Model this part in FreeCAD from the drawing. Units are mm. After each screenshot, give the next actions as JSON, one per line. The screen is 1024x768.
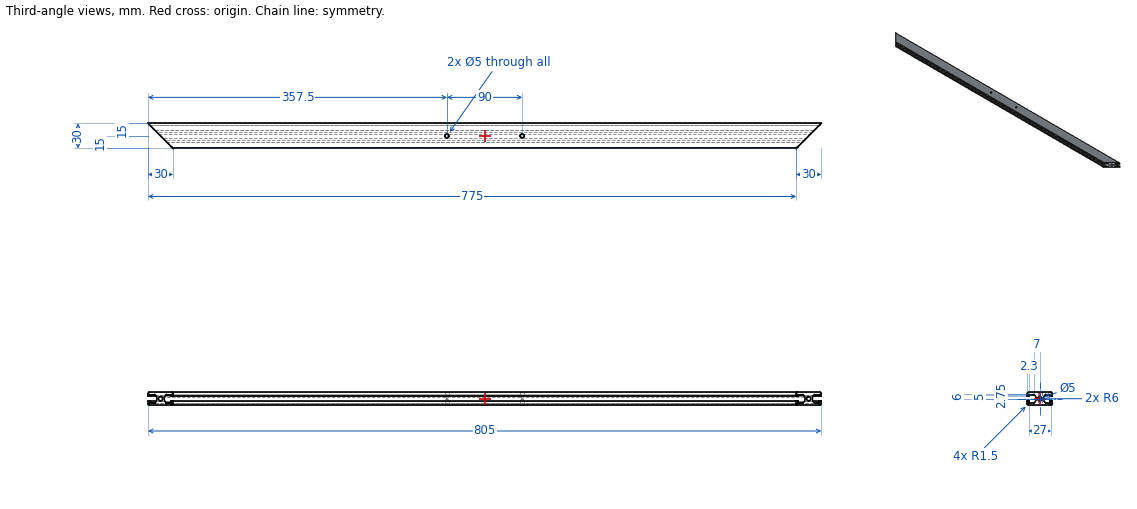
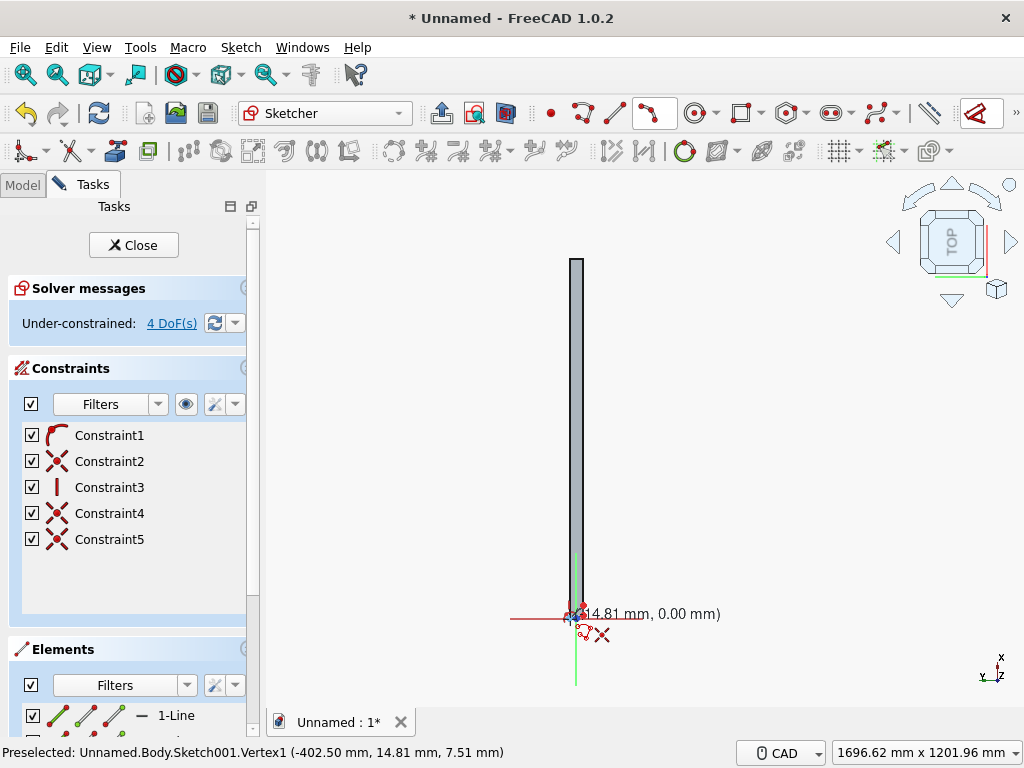
{"action": "scroll", "coordinate": [583, 273], "scroll_direction": "up", "scroll_amount": 5}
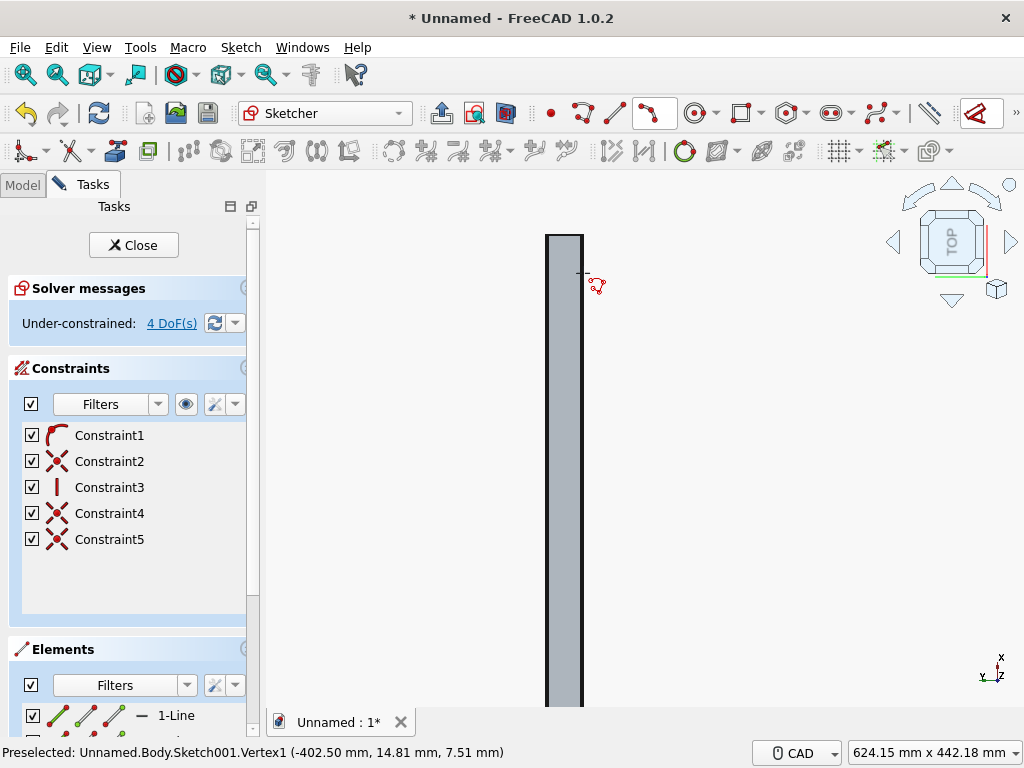
{"action": "left_click", "coordinate": [583, 272]}
{"action": "left_click", "coordinate": [583, 235]}
{"action": "left_click", "coordinate": [546, 235]}
{"action": "left_click", "coordinate": [583, 273]}
{"action": "key", "text": "Escape"}
{"action": "key", "text": "Escape"}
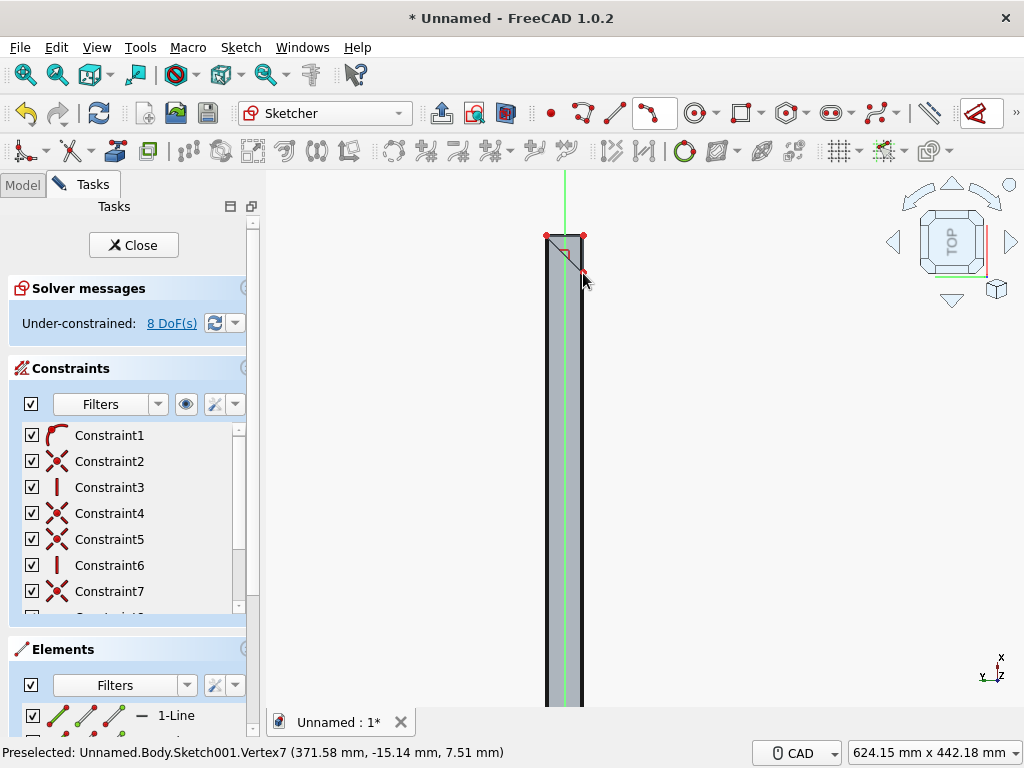
{"action": "scroll", "coordinate": [583, 272], "scroll_direction": "down", "scroll_amount": 5}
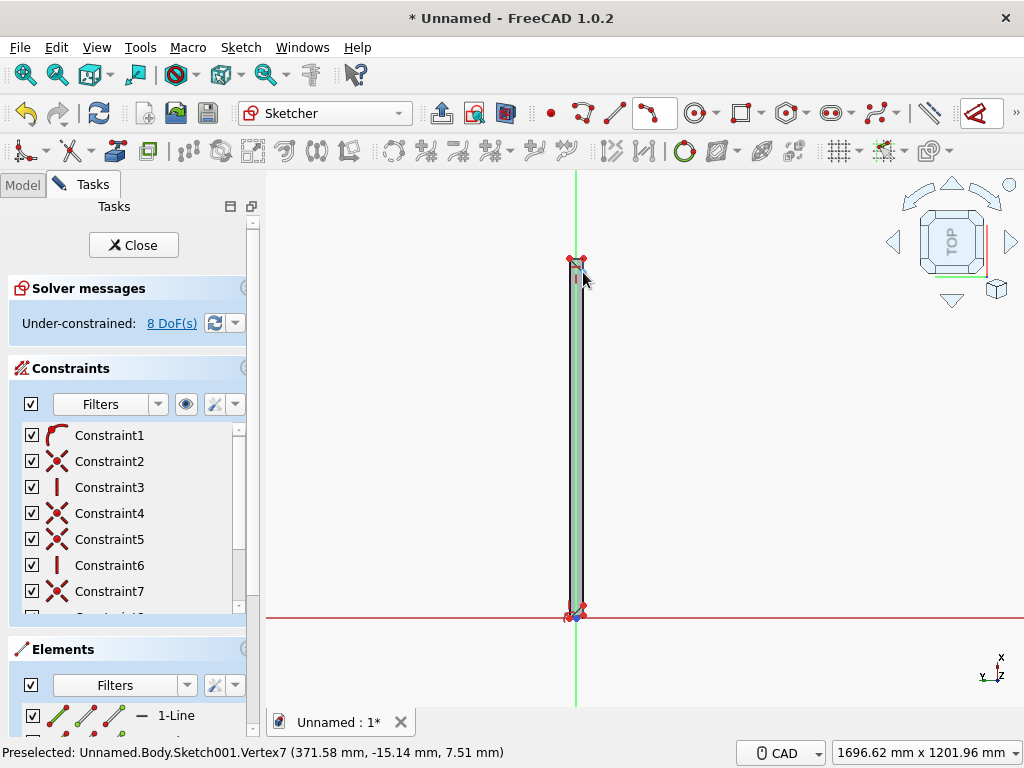
{"action": "scroll", "coordinate": [575, 617], "scroll_direction": "up", "scroll_amount": 8}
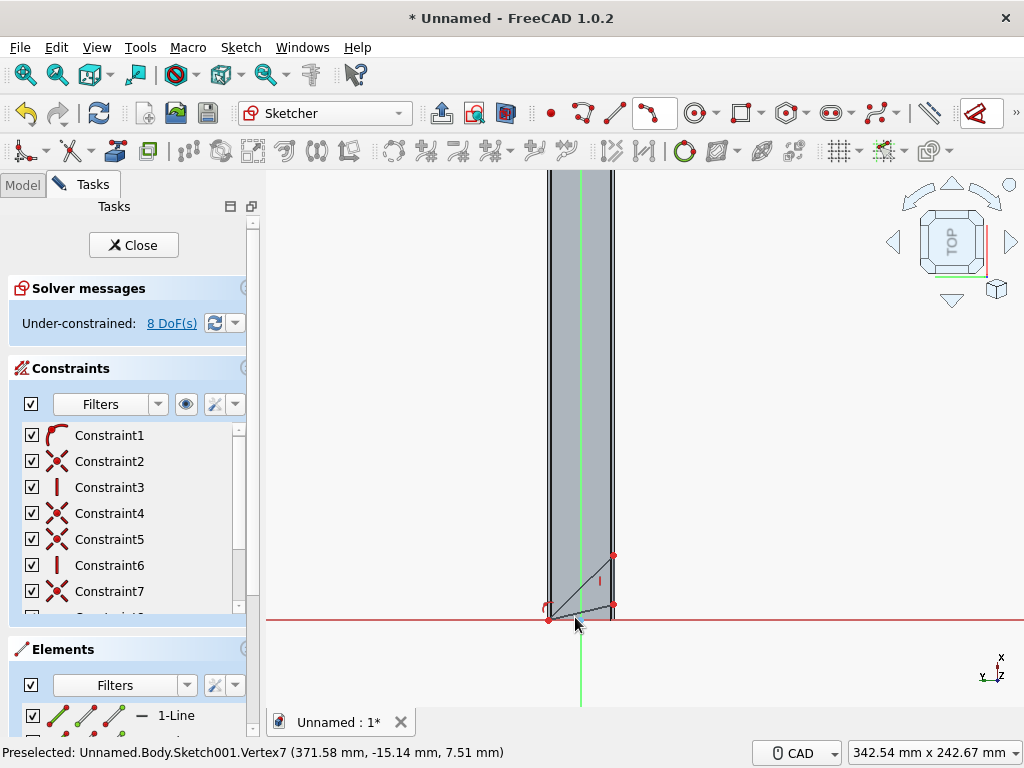
{"action": "left_click", "coordinate": [574, 614]}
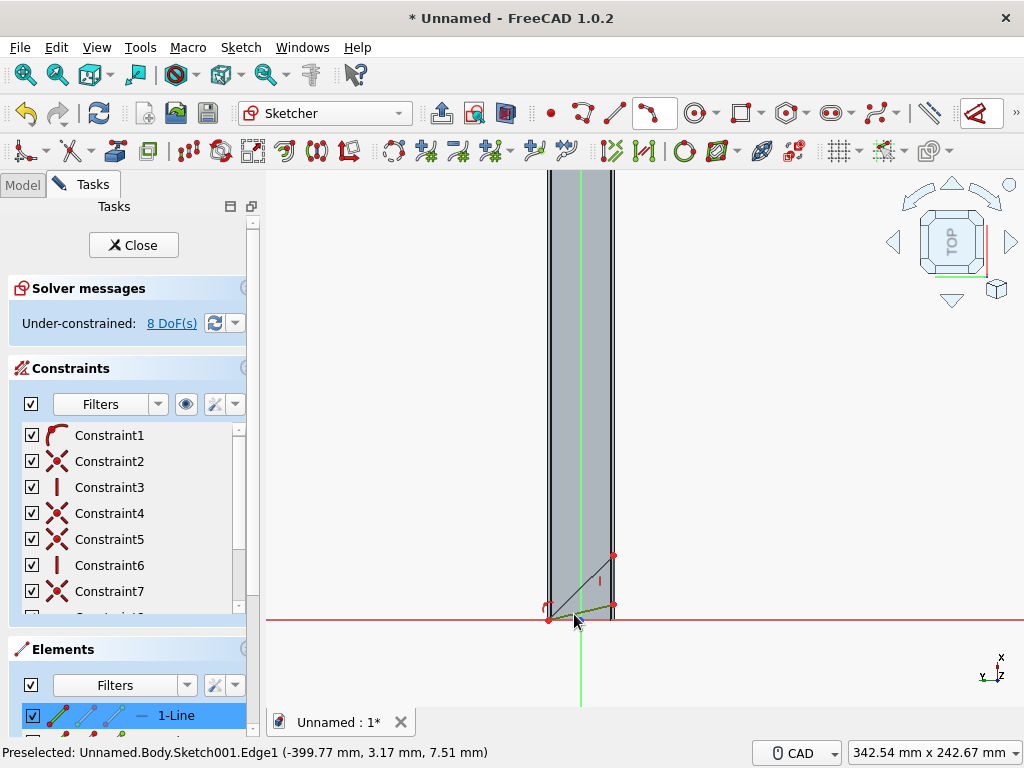
{"action": "key", "text": "h"}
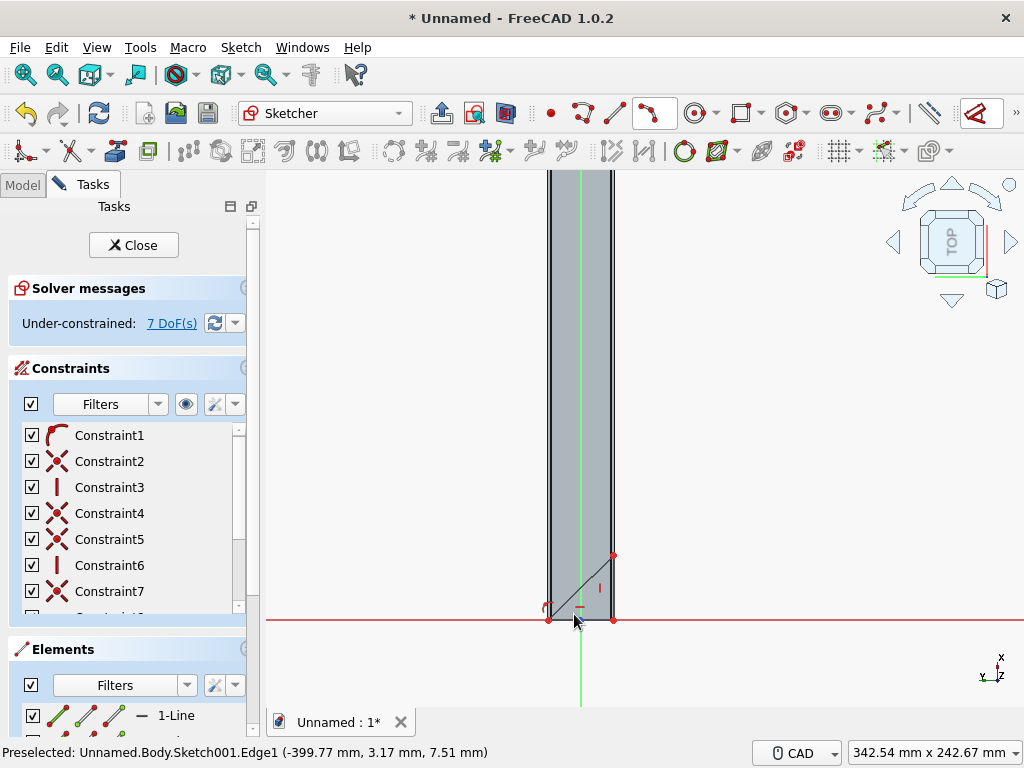
{"action": "left_click", "coordinate": [568, 620]}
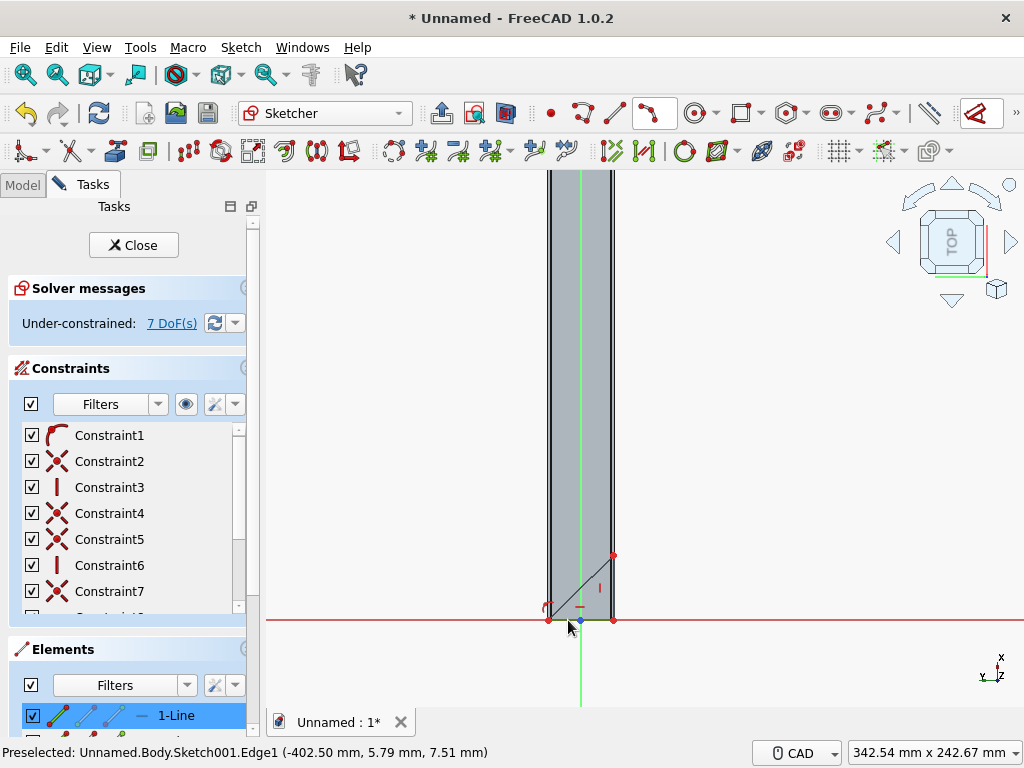
{"action": "left_click", "coordinate": [998, 114]}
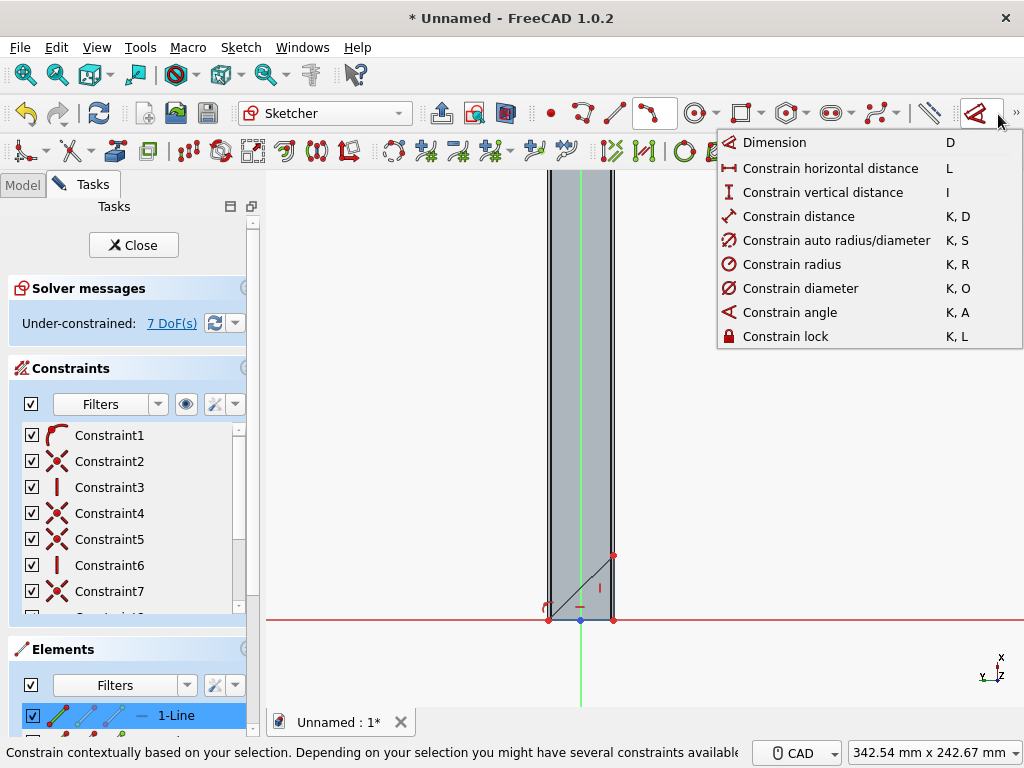
{"action": "left_click", "coordinate": [870, 168]}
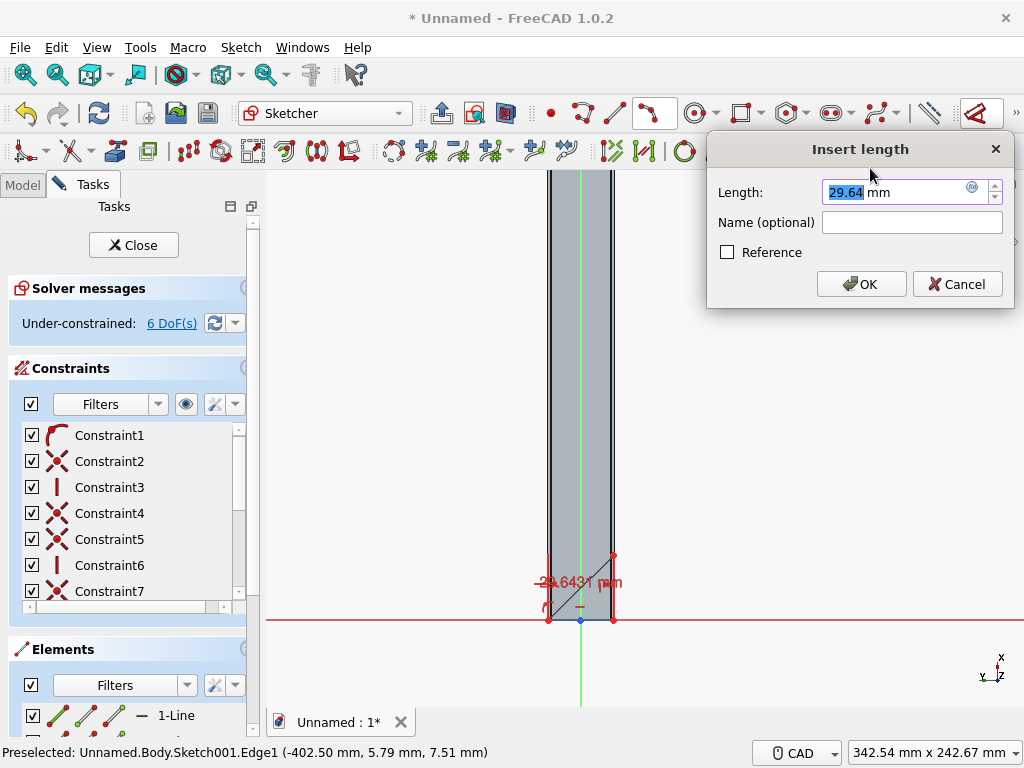
{"action": "type", "text": "30"}
{"action": "key", "text": "Return"}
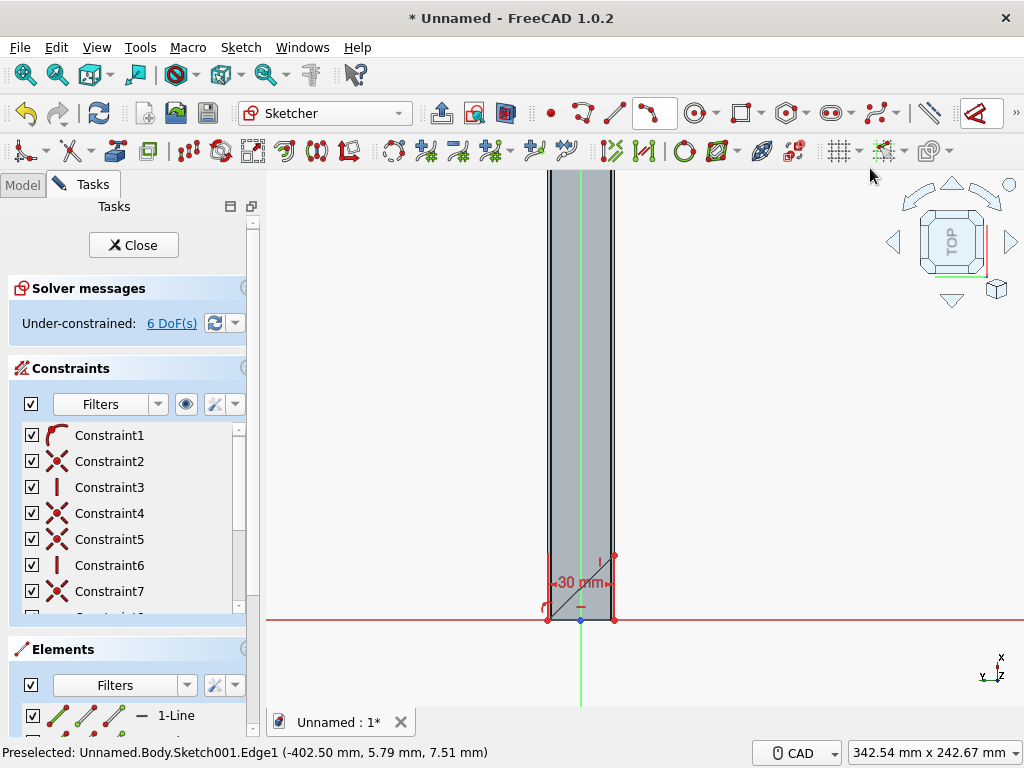
{"action": "left_click", "coordinate": [614, 601]}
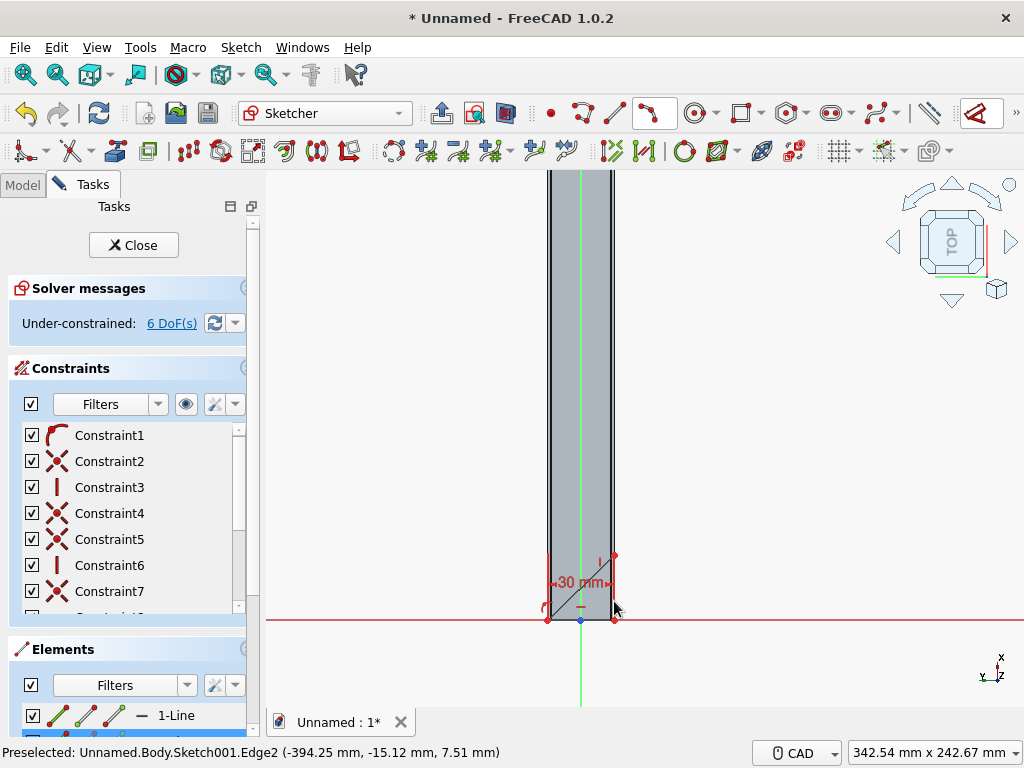
{"action": "key", "text": "i"}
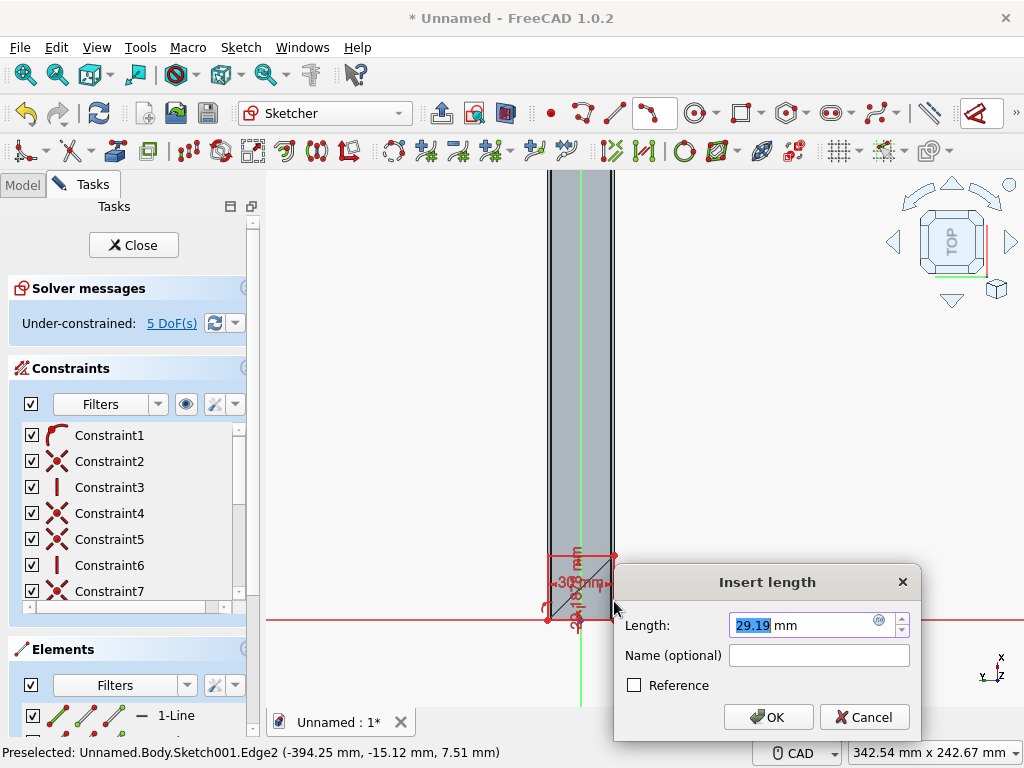
{"action": "type", "text": "30"}
{"action": "key", "text": "Return"}